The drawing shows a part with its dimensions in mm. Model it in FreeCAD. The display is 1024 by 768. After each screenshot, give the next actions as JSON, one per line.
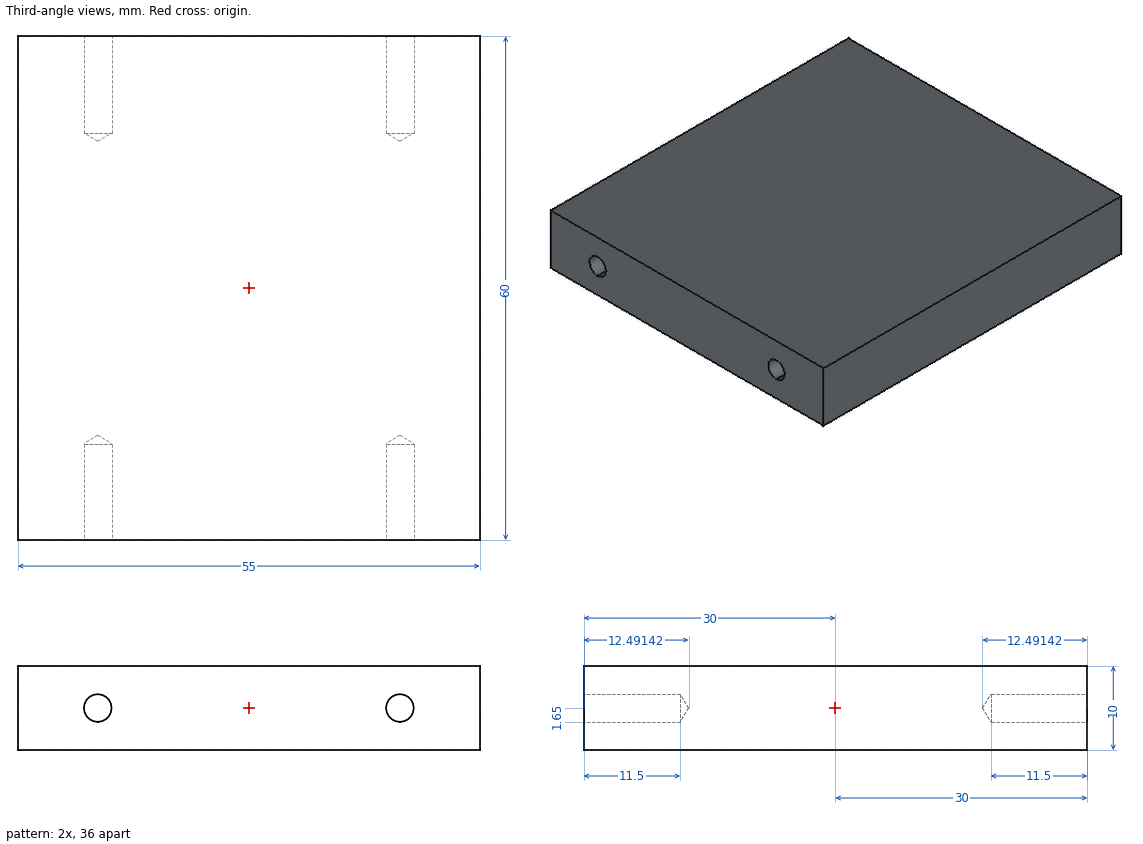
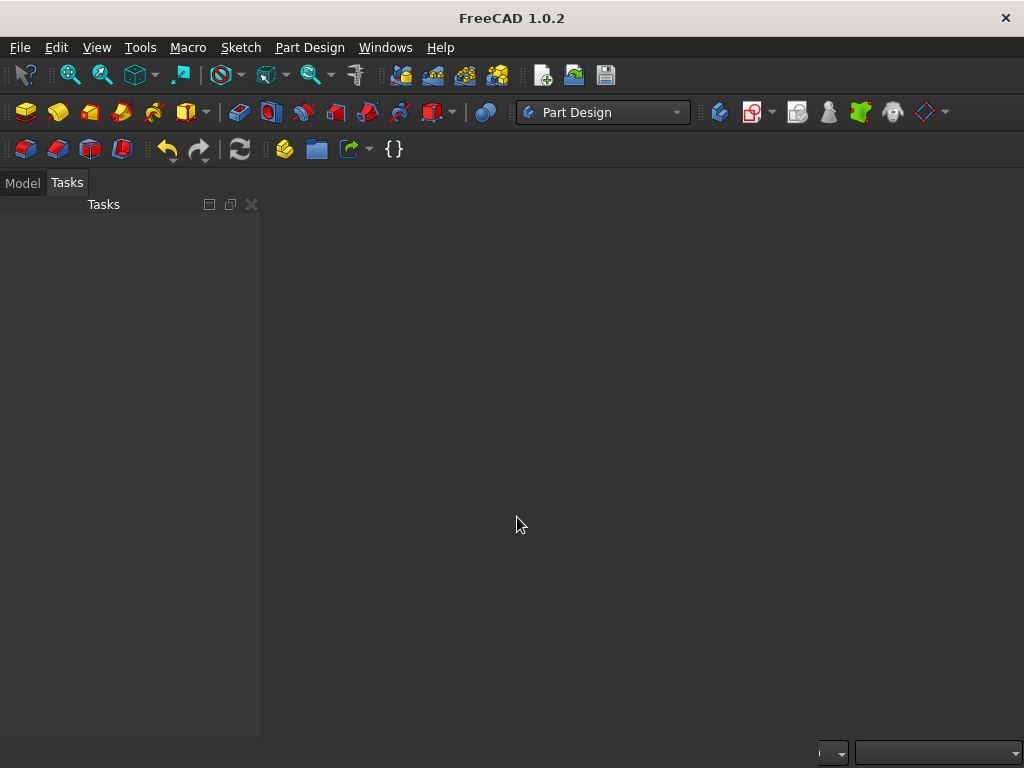
{"action": "key", "text": "ctrl+n"}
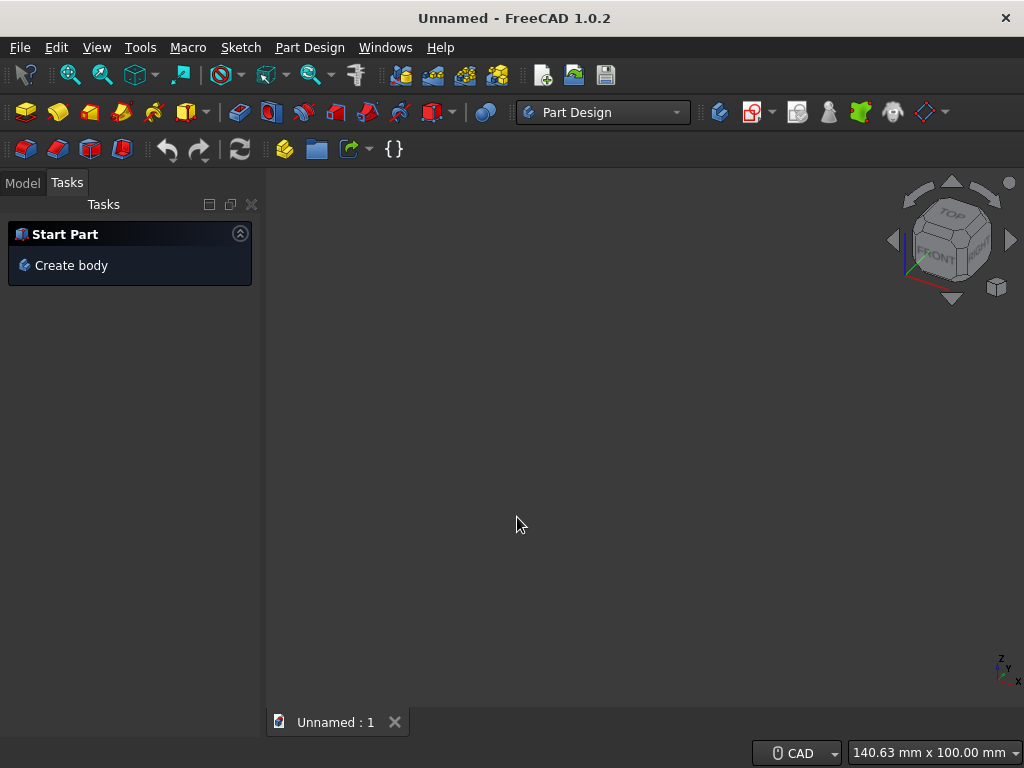
{"action": "left_click", "coordinate": [752, 112]}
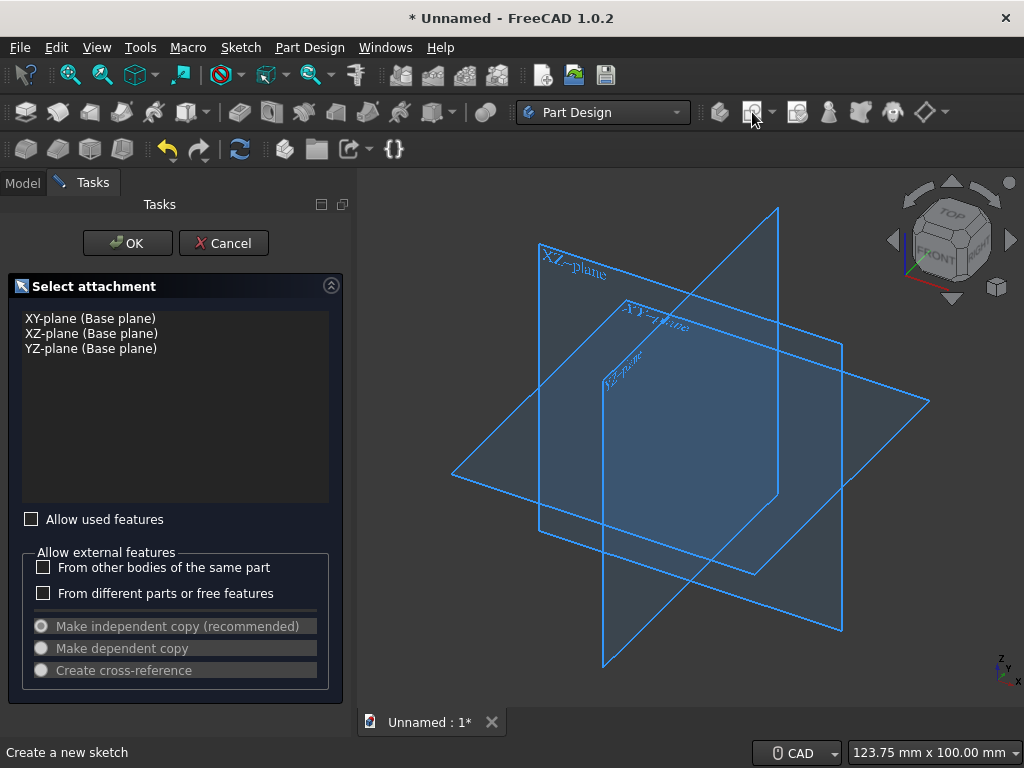
{"action": "left_click", "coordinate": [82, 318]}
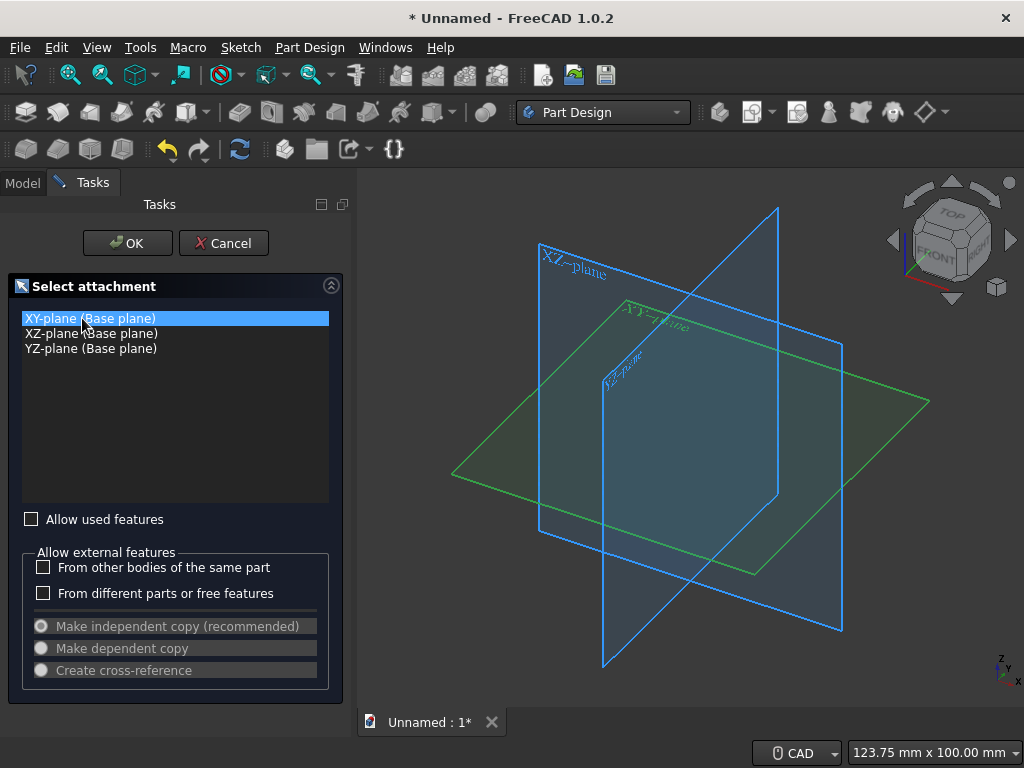
{"action": "left_click", "coordinate": [128, 243]}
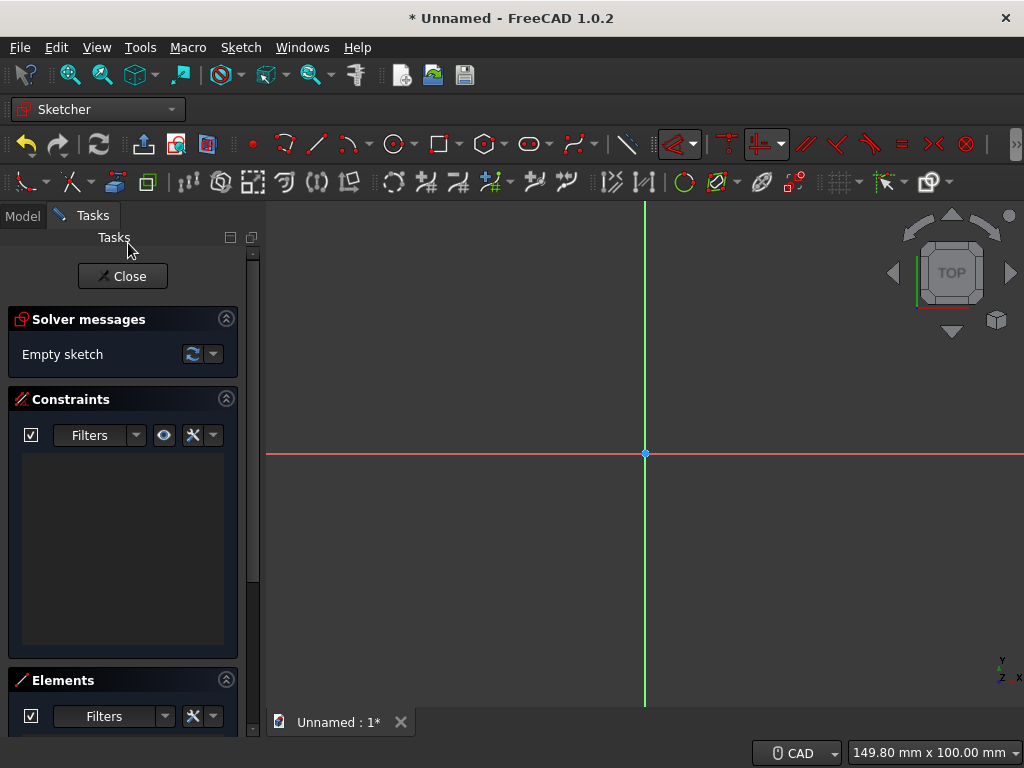
{"action": "key", "text": "g v"}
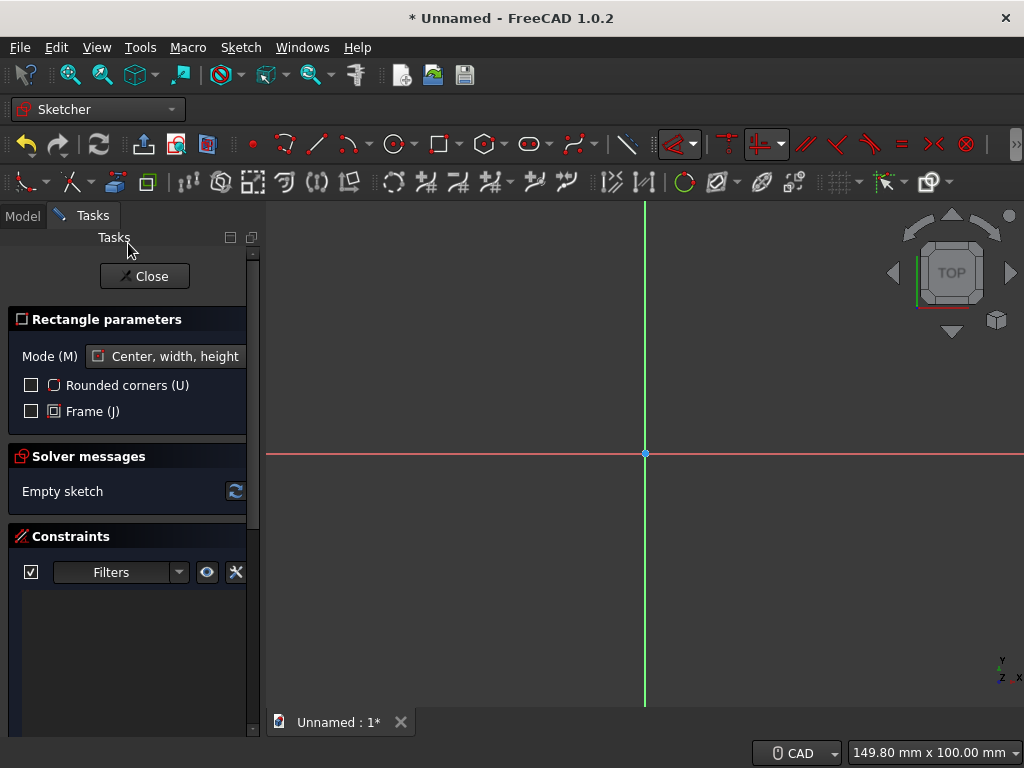
{"action": "left_click", "coordinate": [645, 454]}
{"action": "left_click", "coordinate": [784, 302]}
{"action": "key", "text": "Escape"}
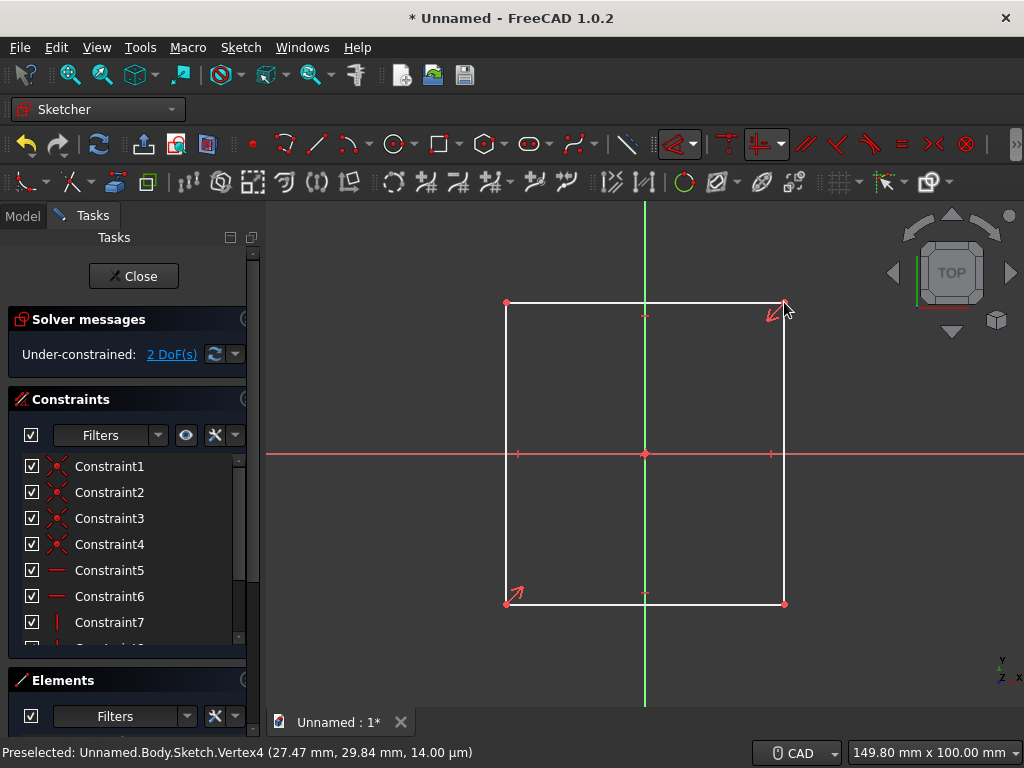
{"action": "key", "text": "d"}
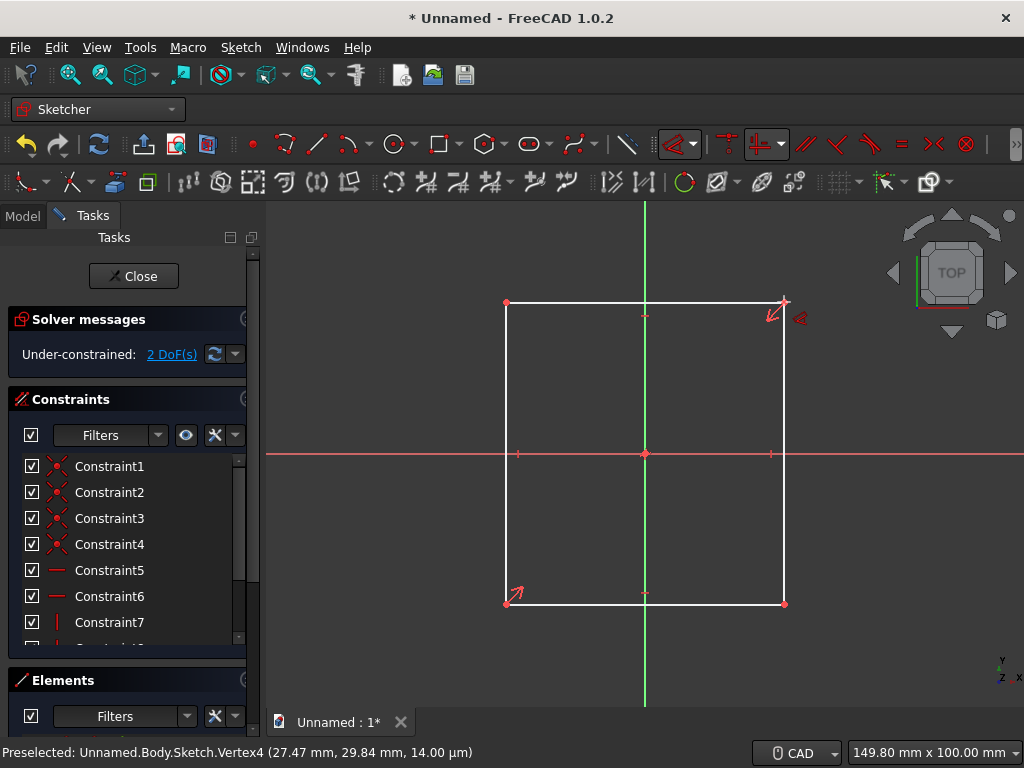
{"action": "left_click", "coordinate": [589, 605]}
{"action": "left_click", "coordinate": [581, 639]}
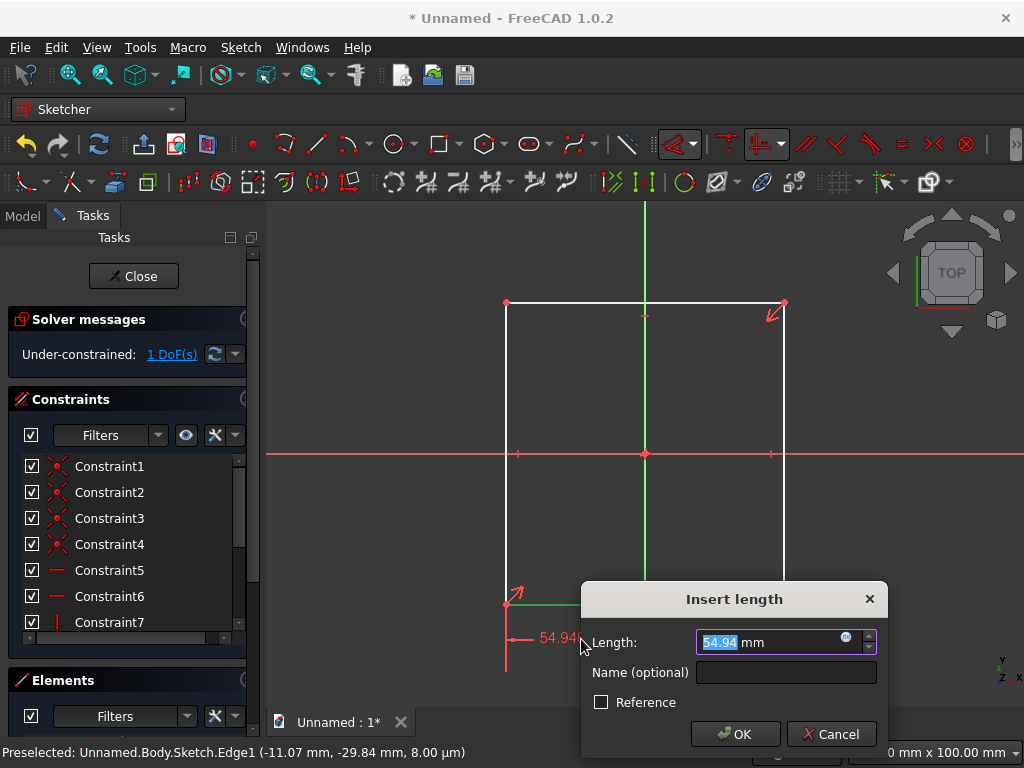
{"action": "type", "text": "55"}
{"action": "key", "text": "Return"}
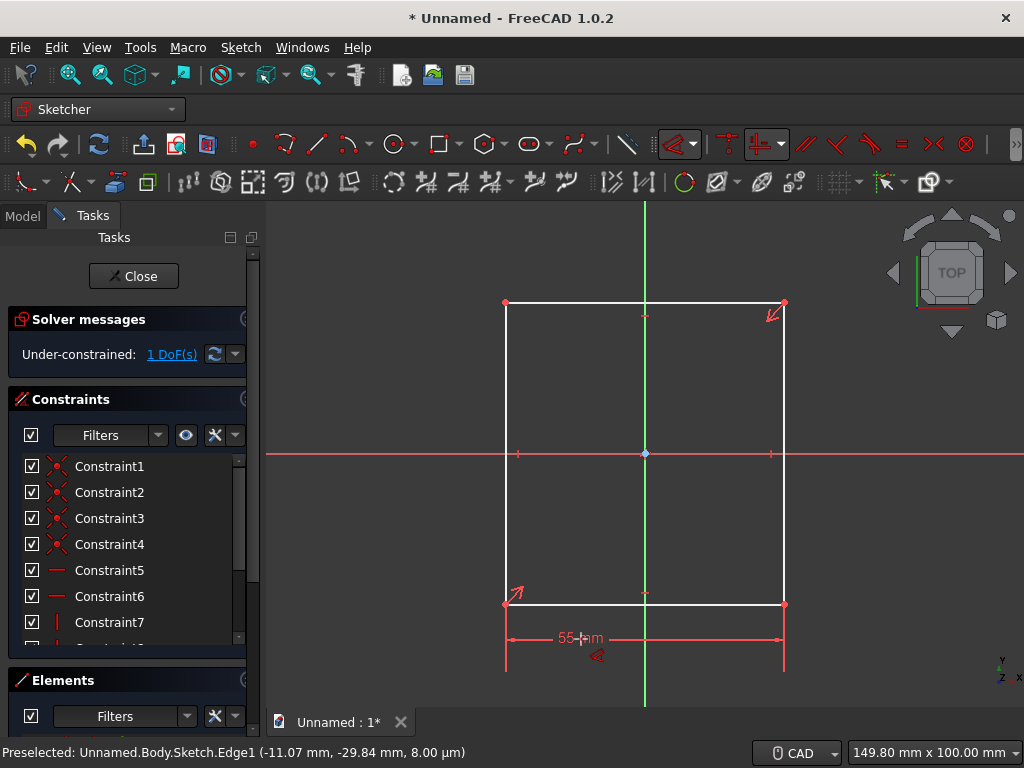
{"action": "left_click", "coordinate": [784, 514]}
{"action": "left_click", "coordinate": [818, 385]}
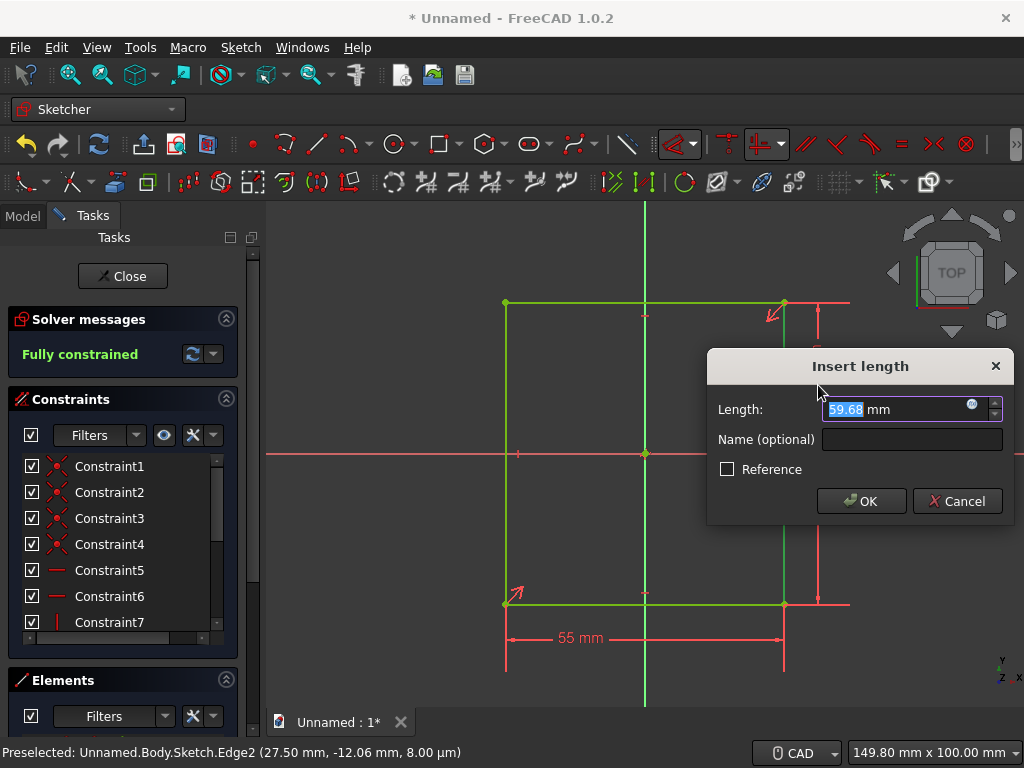
{"action": "type", "text": "60"}
{"action": "key", "text": "Return"}
{"action": "key", "text": "Escape"}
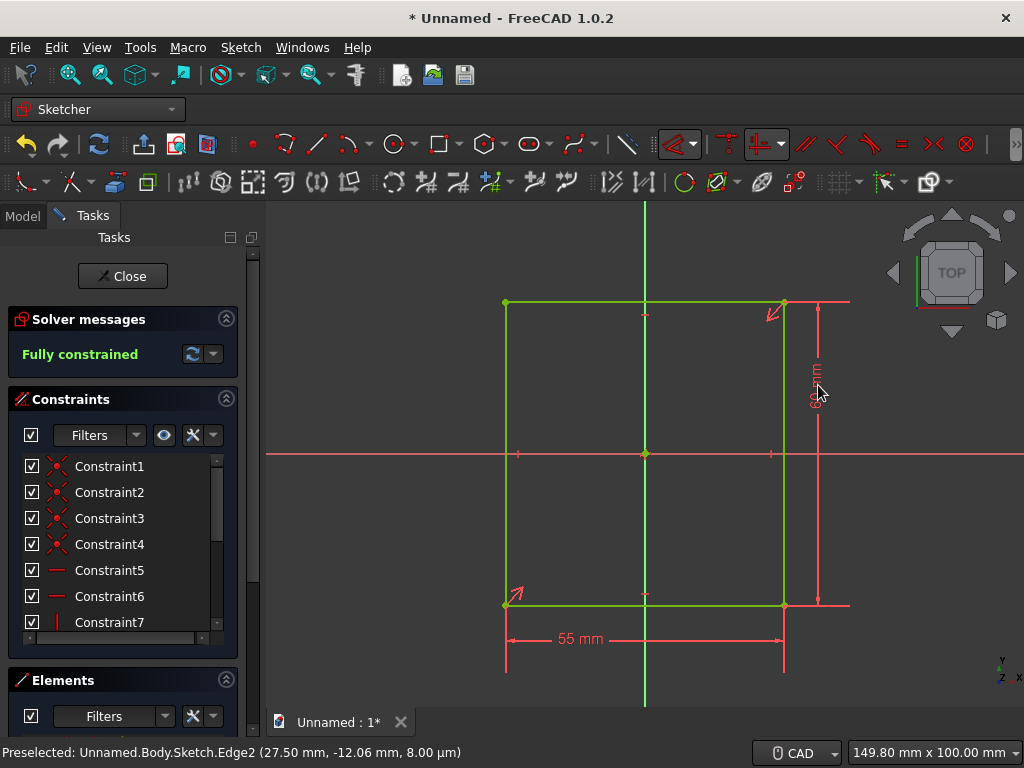
{"action": "left_click", "coordinate": [123, 276]}